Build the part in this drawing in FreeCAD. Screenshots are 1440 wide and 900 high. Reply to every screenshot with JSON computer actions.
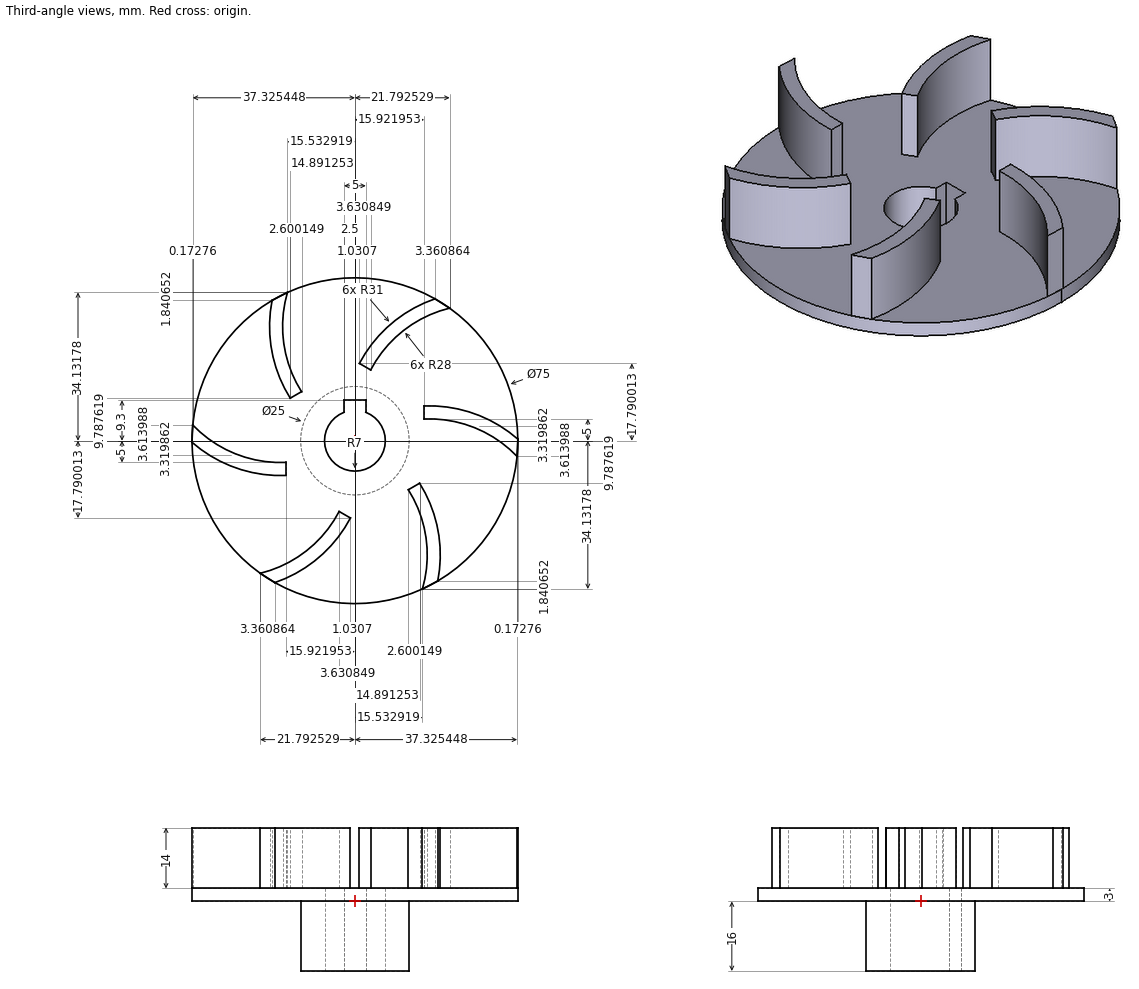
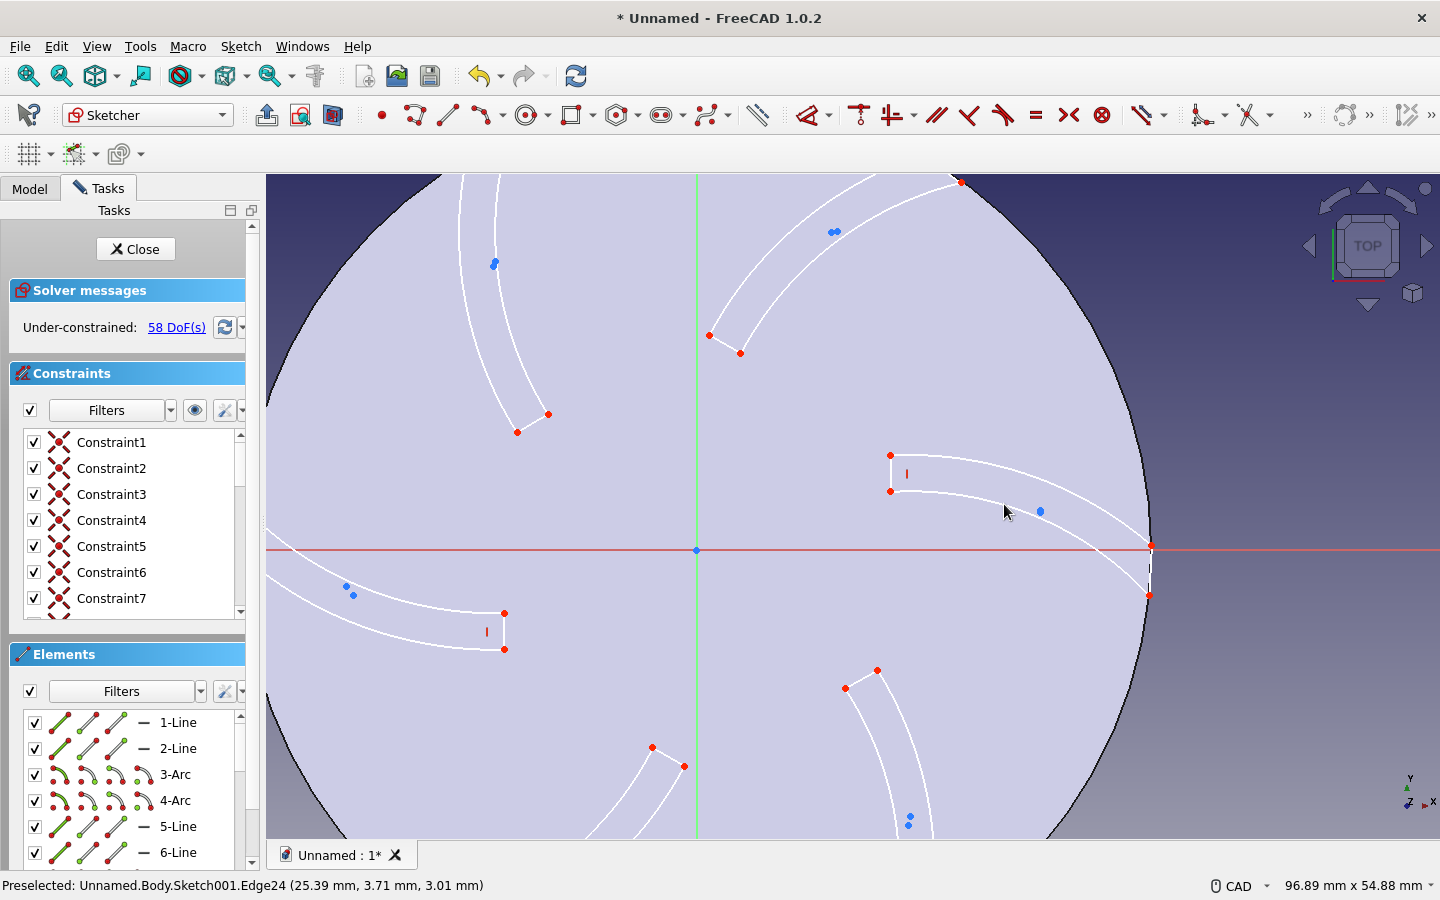
{"action": "left_click", "coordinate": [758, 265]}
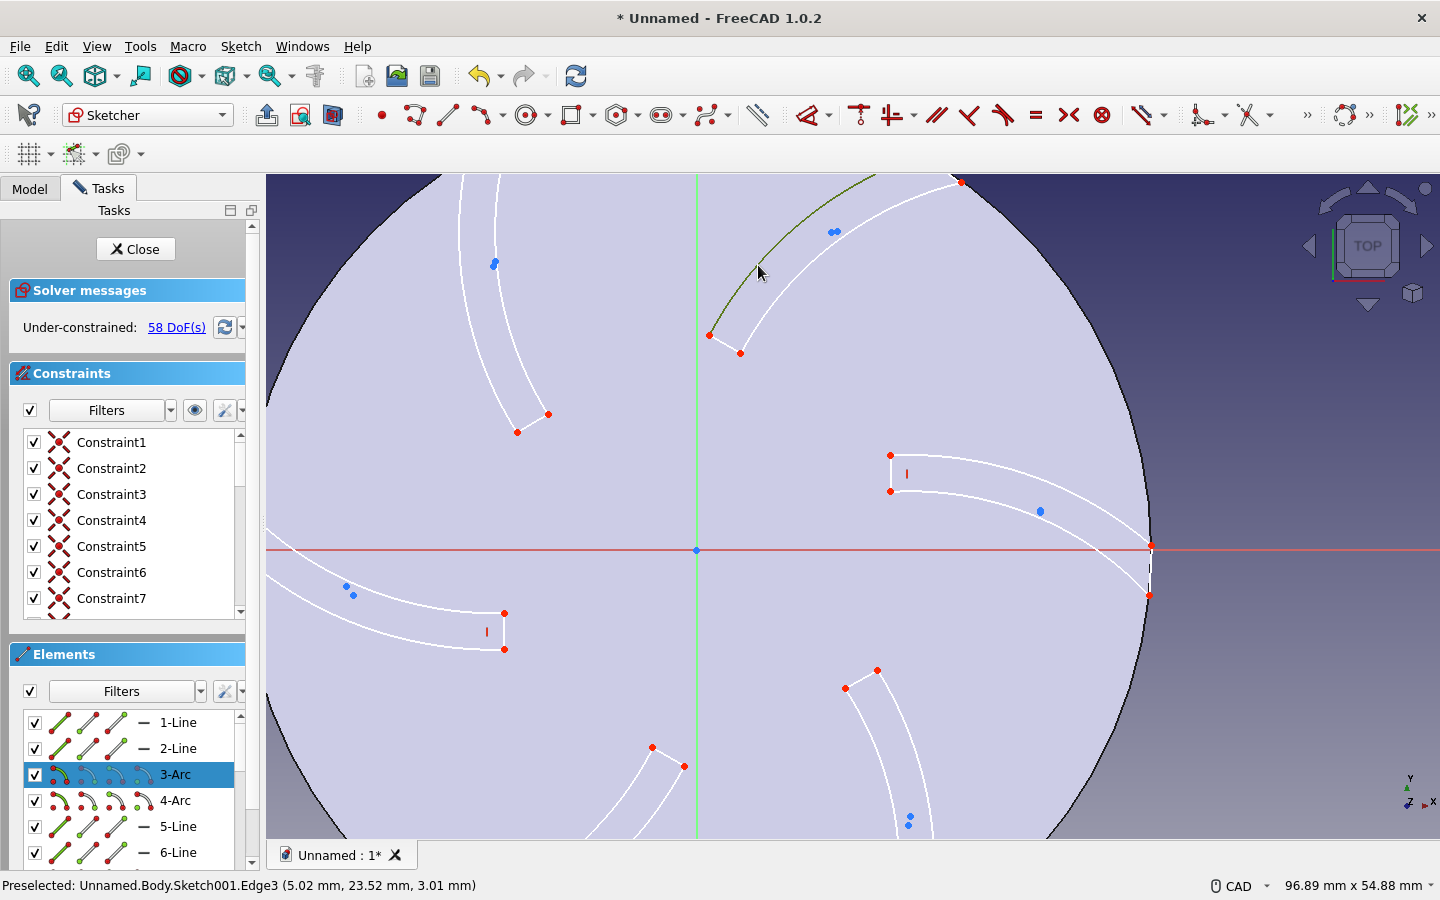
{"action": "left_click", "coordinate": [881, 213]}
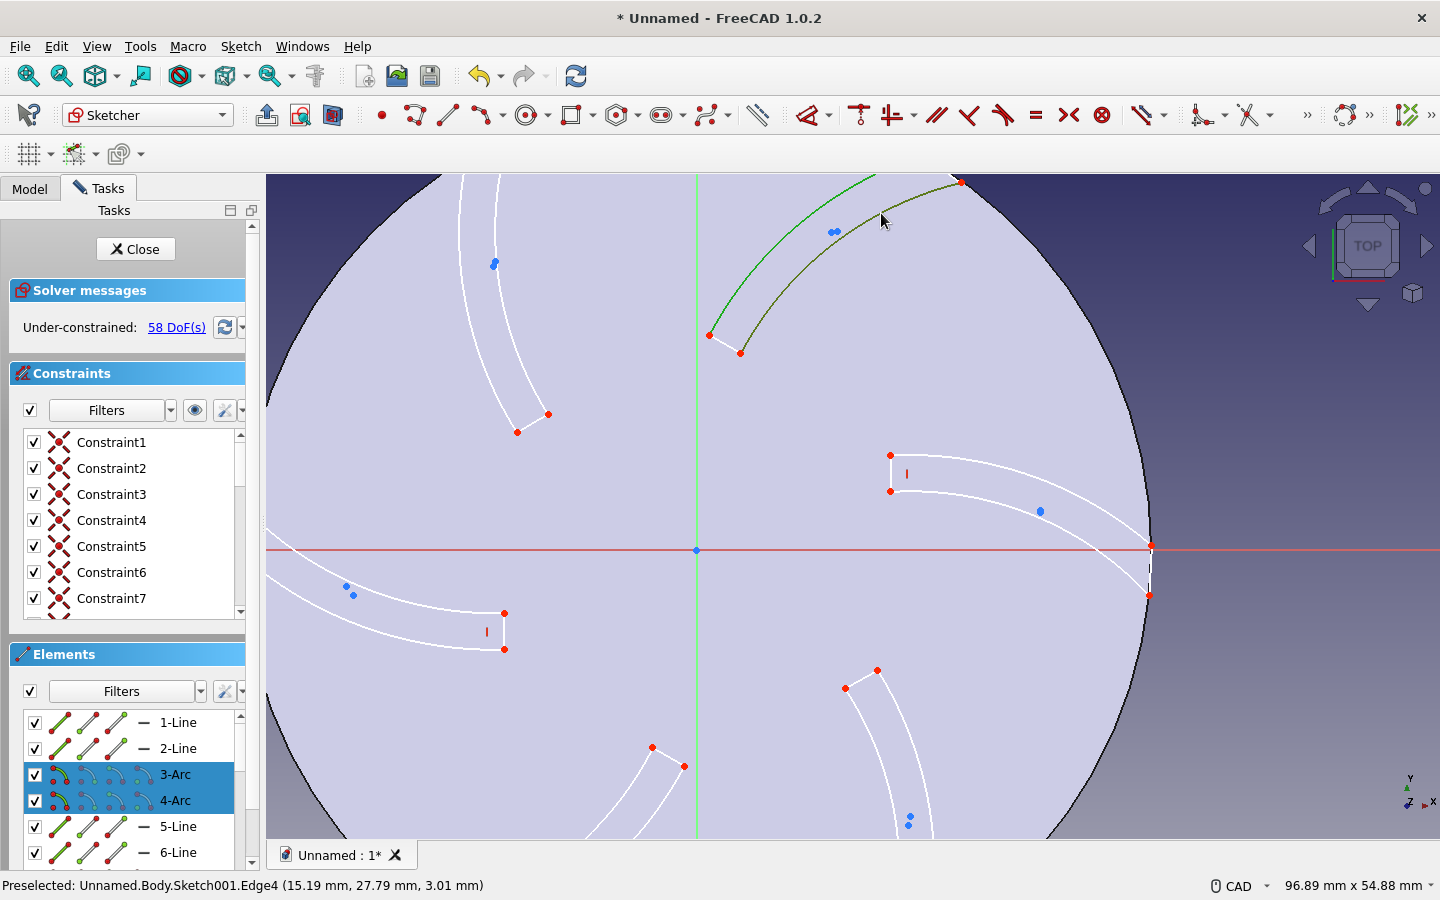
{"action": "key", "text": "c"}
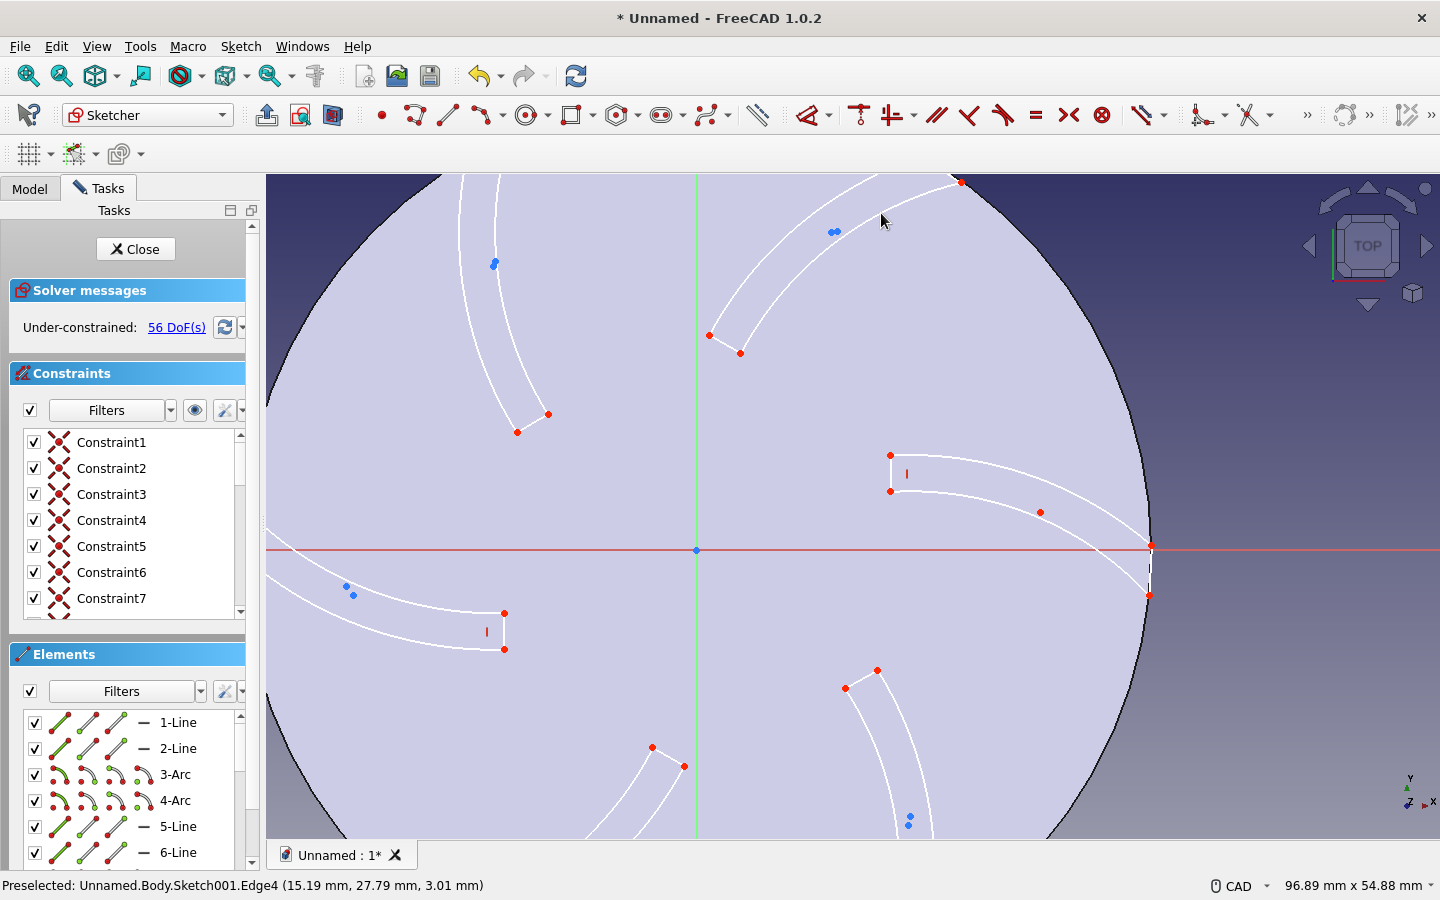
{"action": "left_click", "coordinate": [459, 245]}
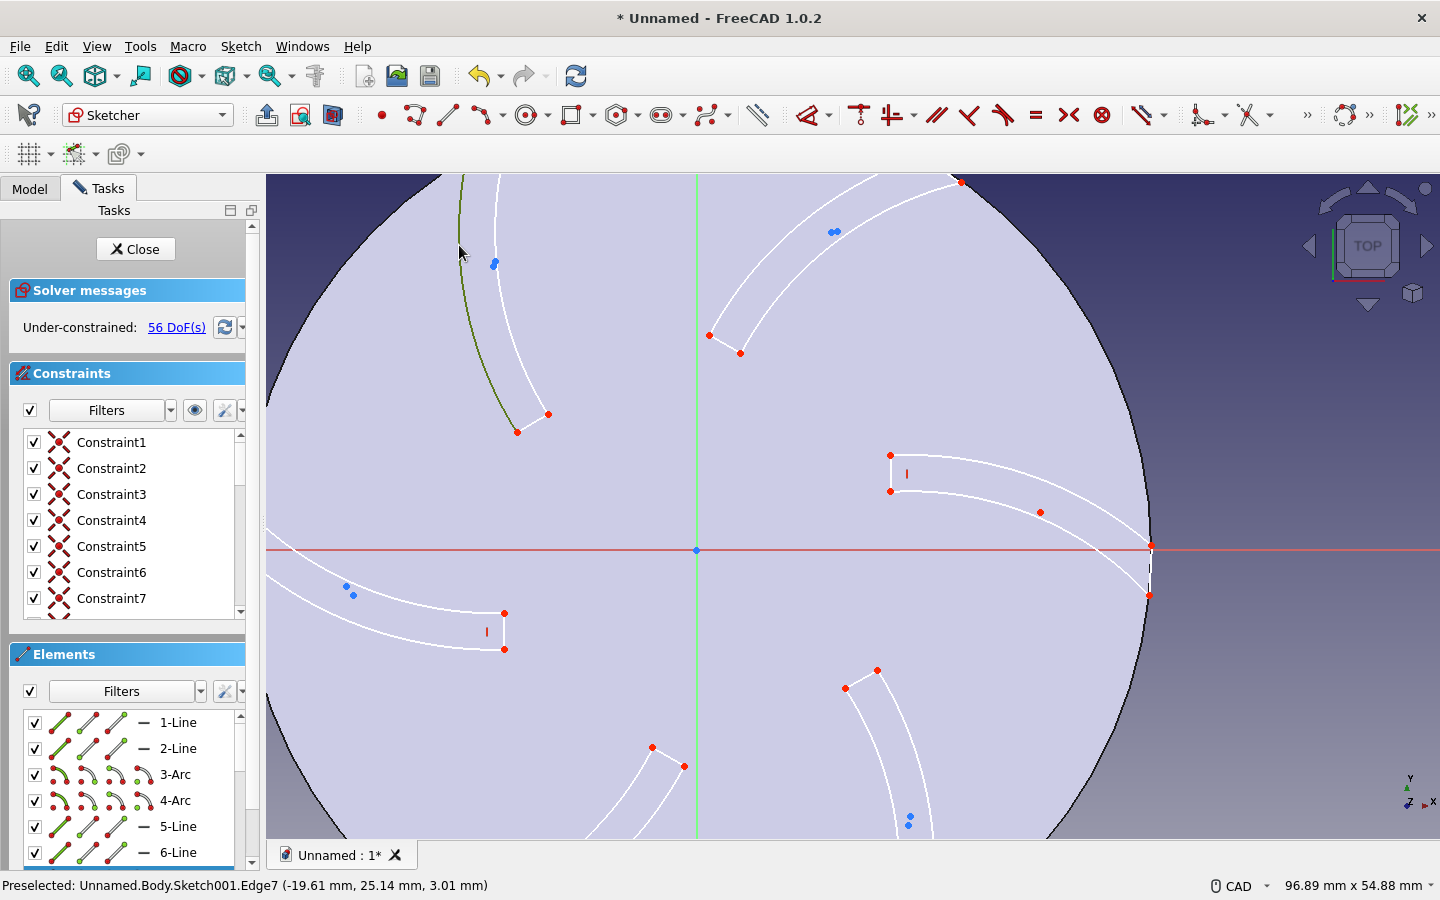
{"action": "left_click", "coordinate": [495, 224]}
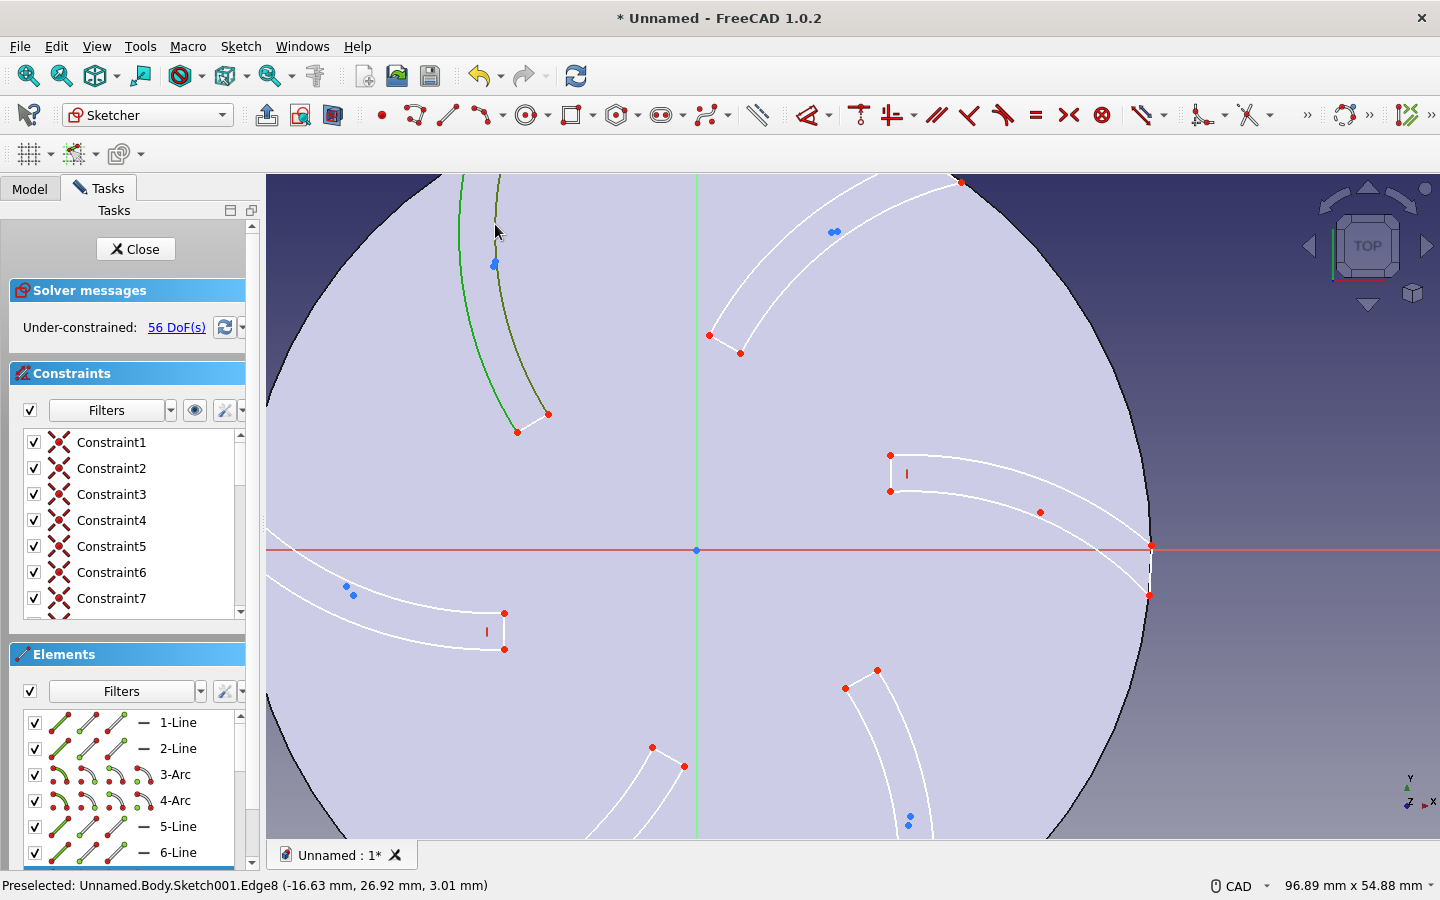
{"action": "key", "text": "c"}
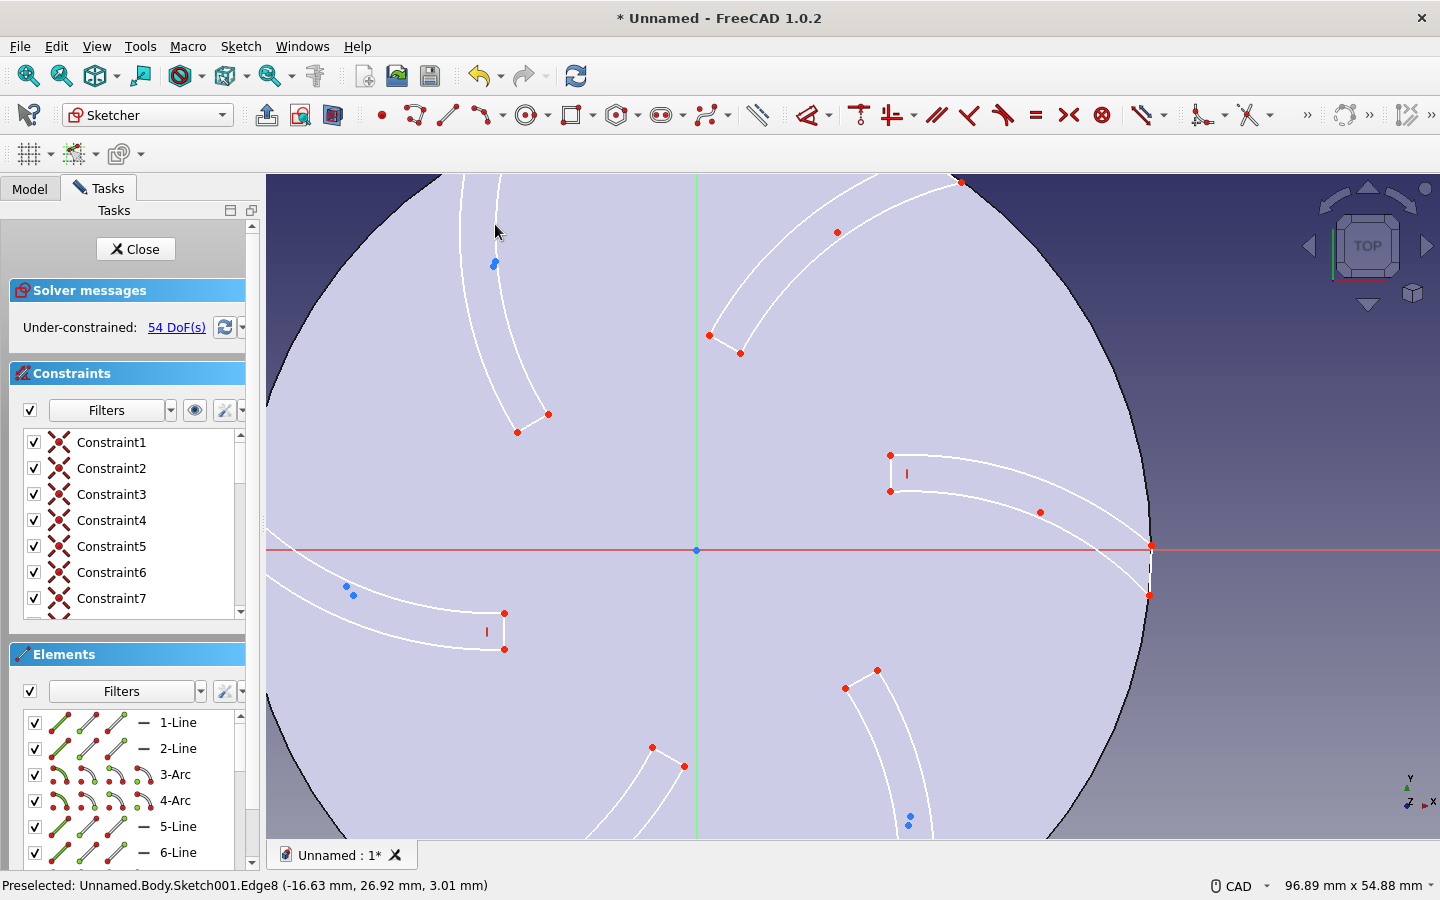
{"action": "left_click", "coordinate": [312, 604]}